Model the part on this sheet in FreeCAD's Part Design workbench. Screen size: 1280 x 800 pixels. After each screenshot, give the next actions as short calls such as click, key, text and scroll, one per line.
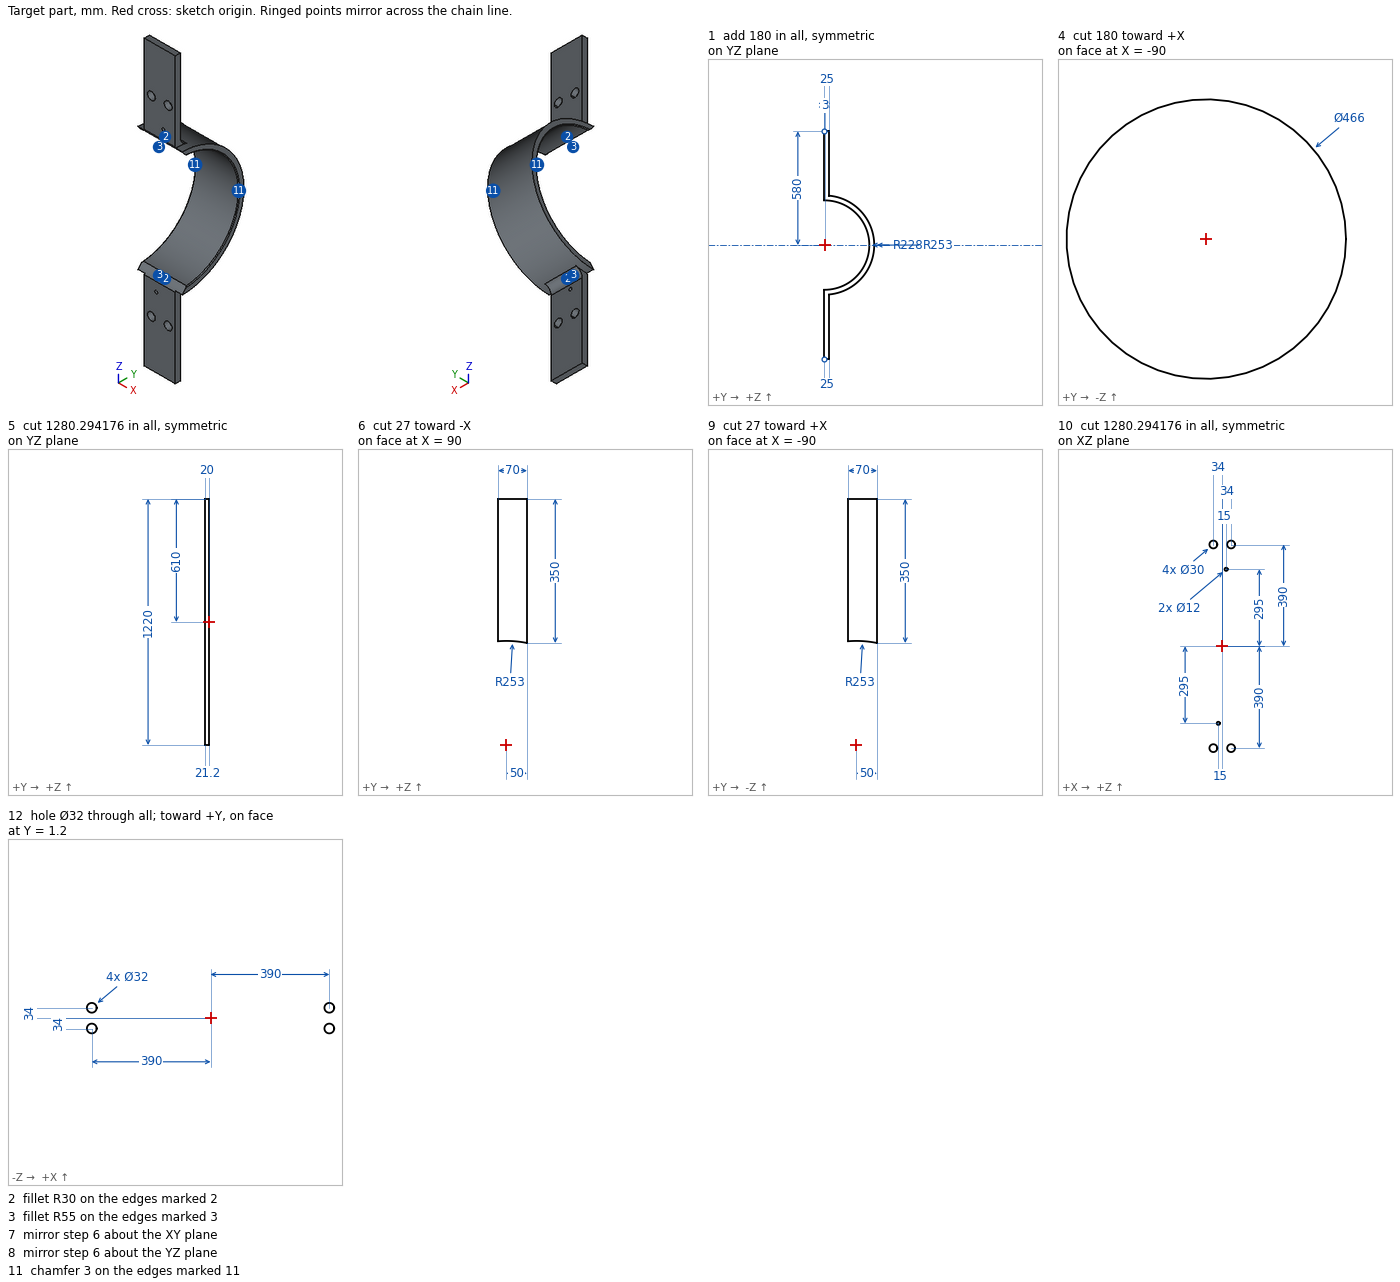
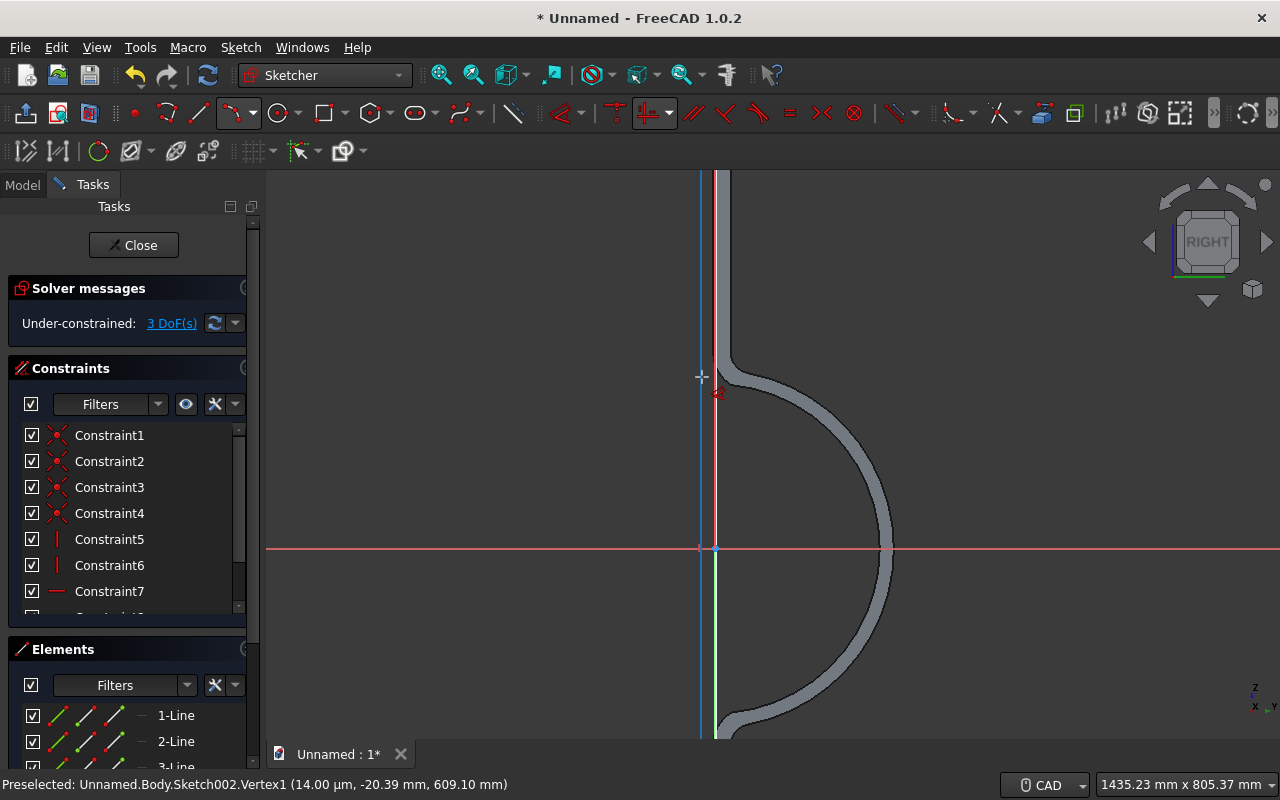
click(701, 377)
click(667, 454)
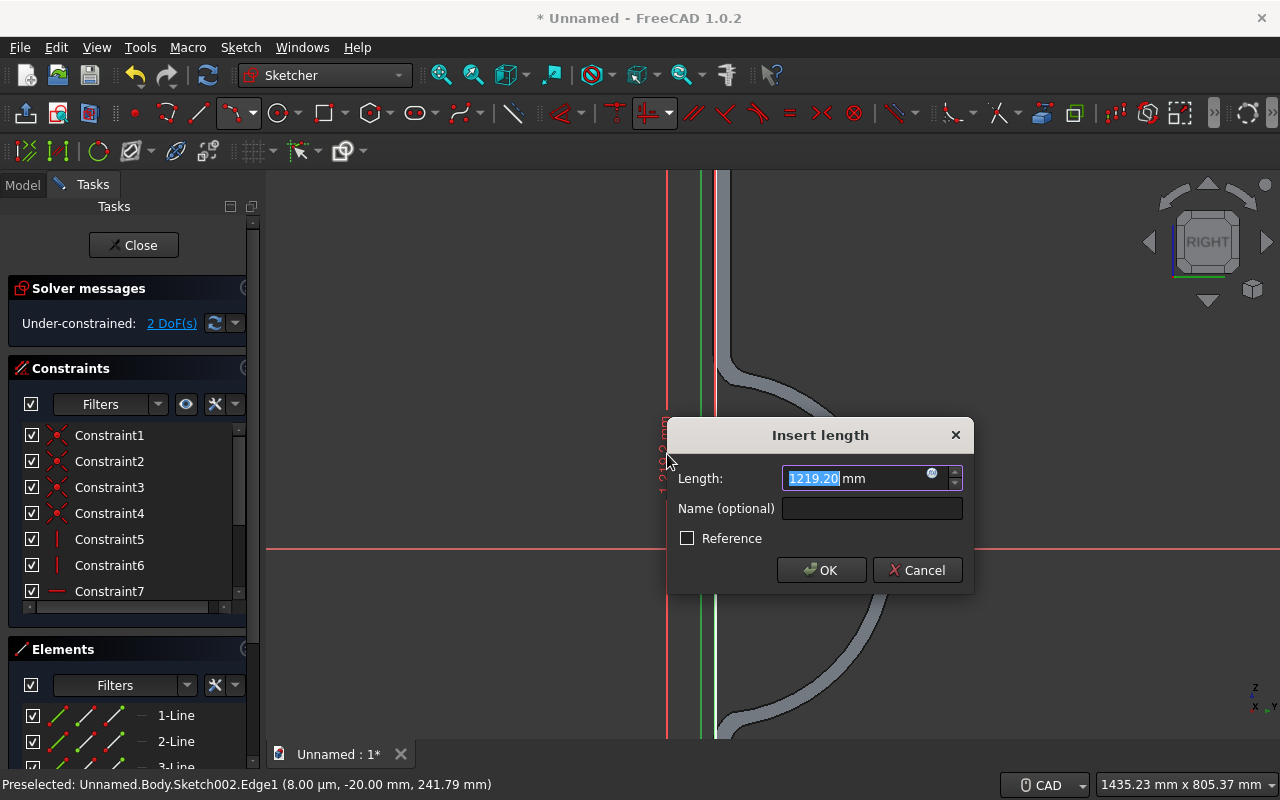
text(1220)
key(Return)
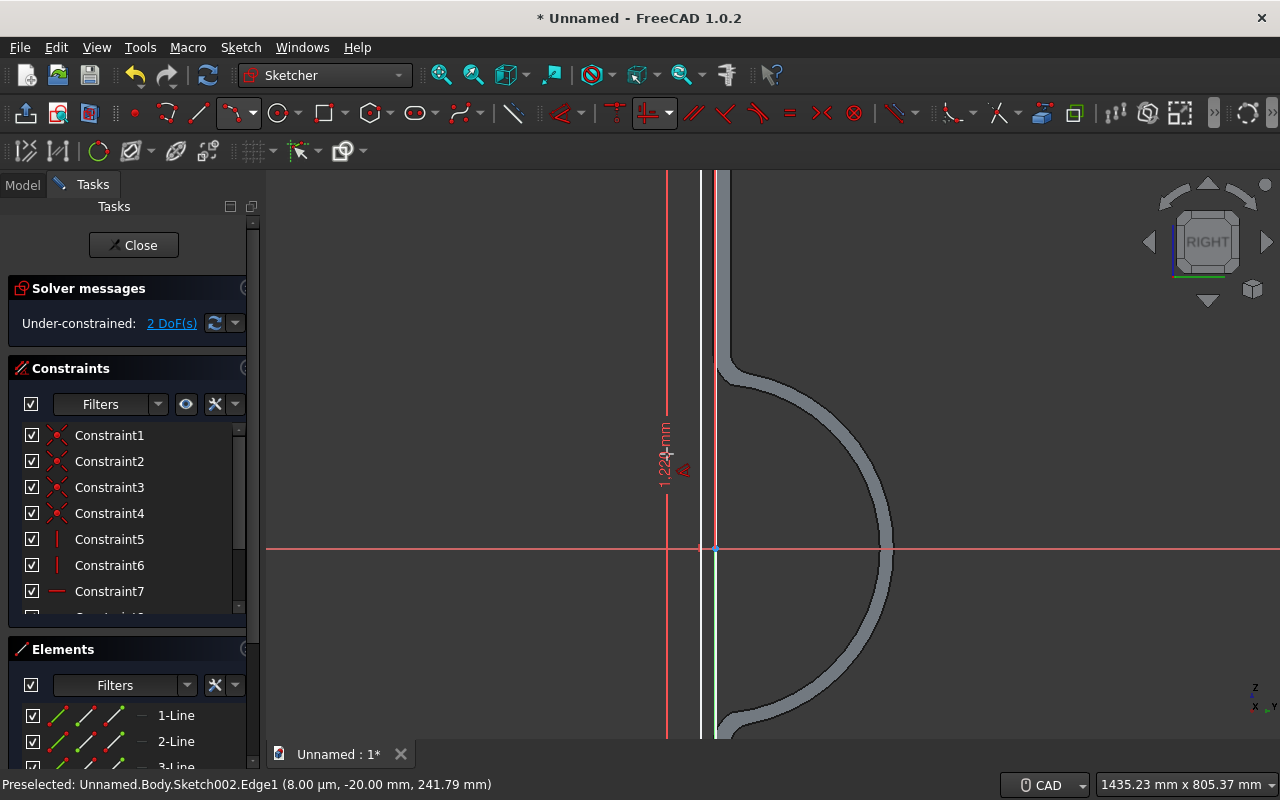
scroll(701, 378, down, 4)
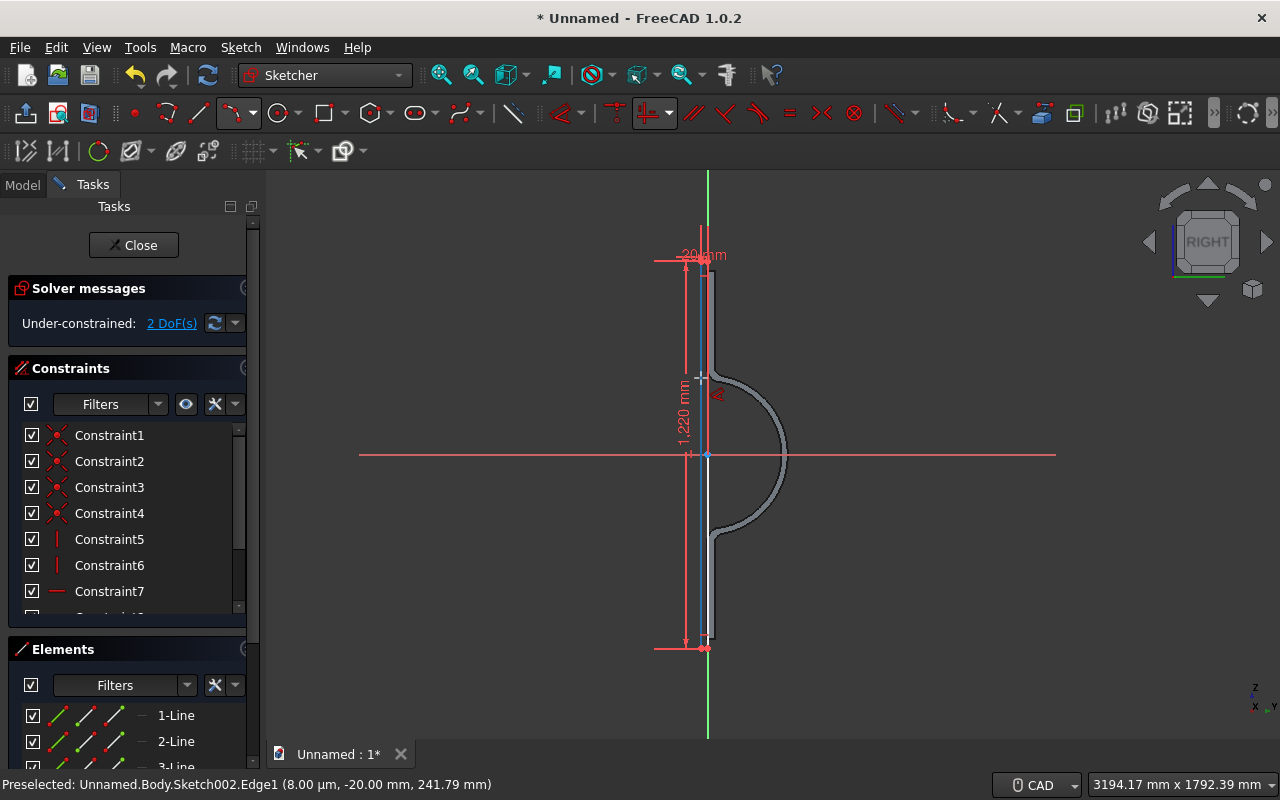
scroll(705, 649, up, 9)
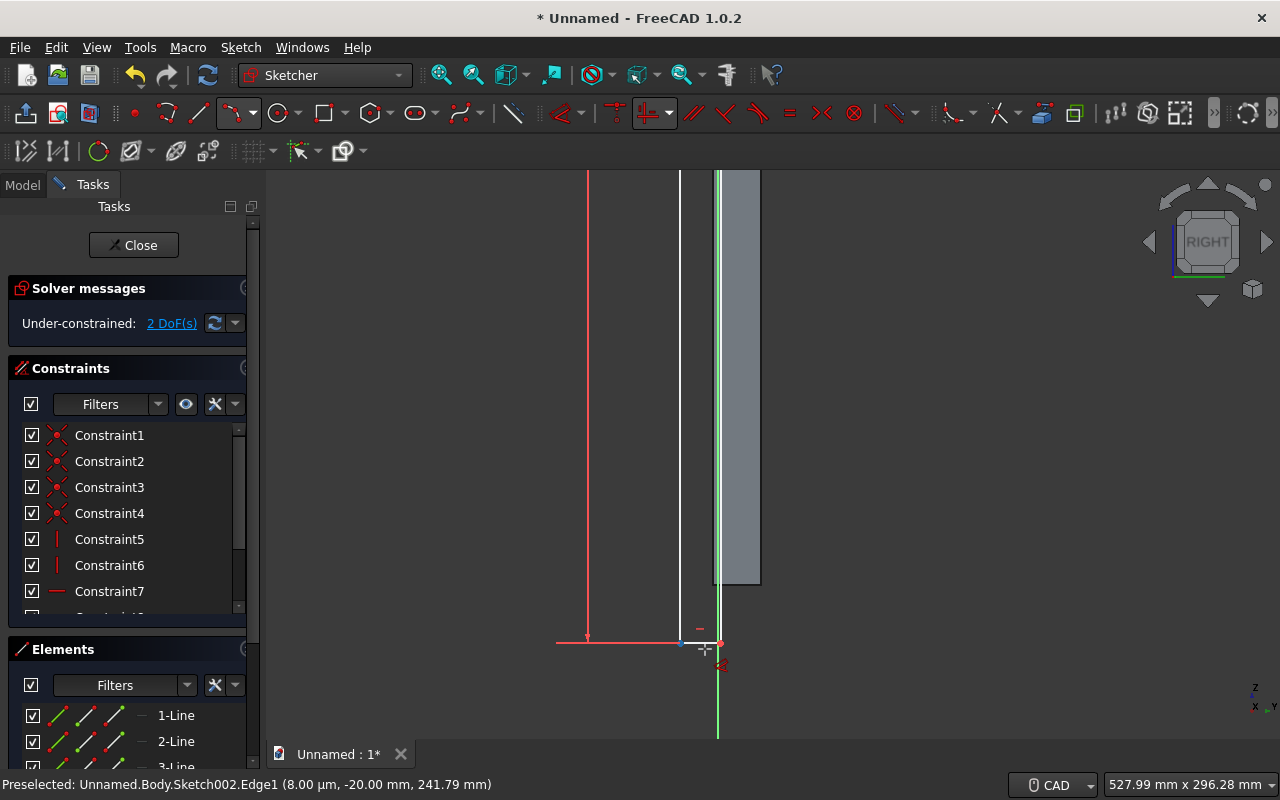
click(700, 643)
click(700, 677)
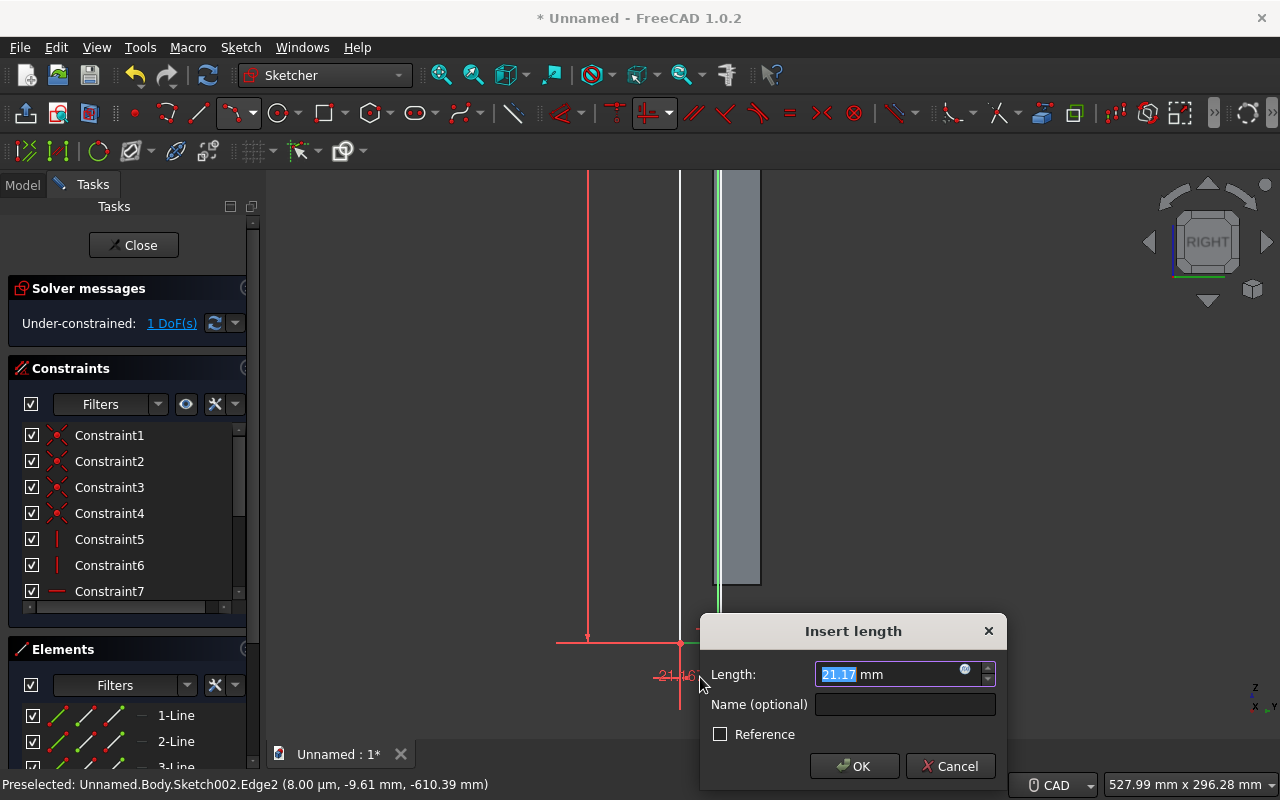
text(21.2)
key(Return)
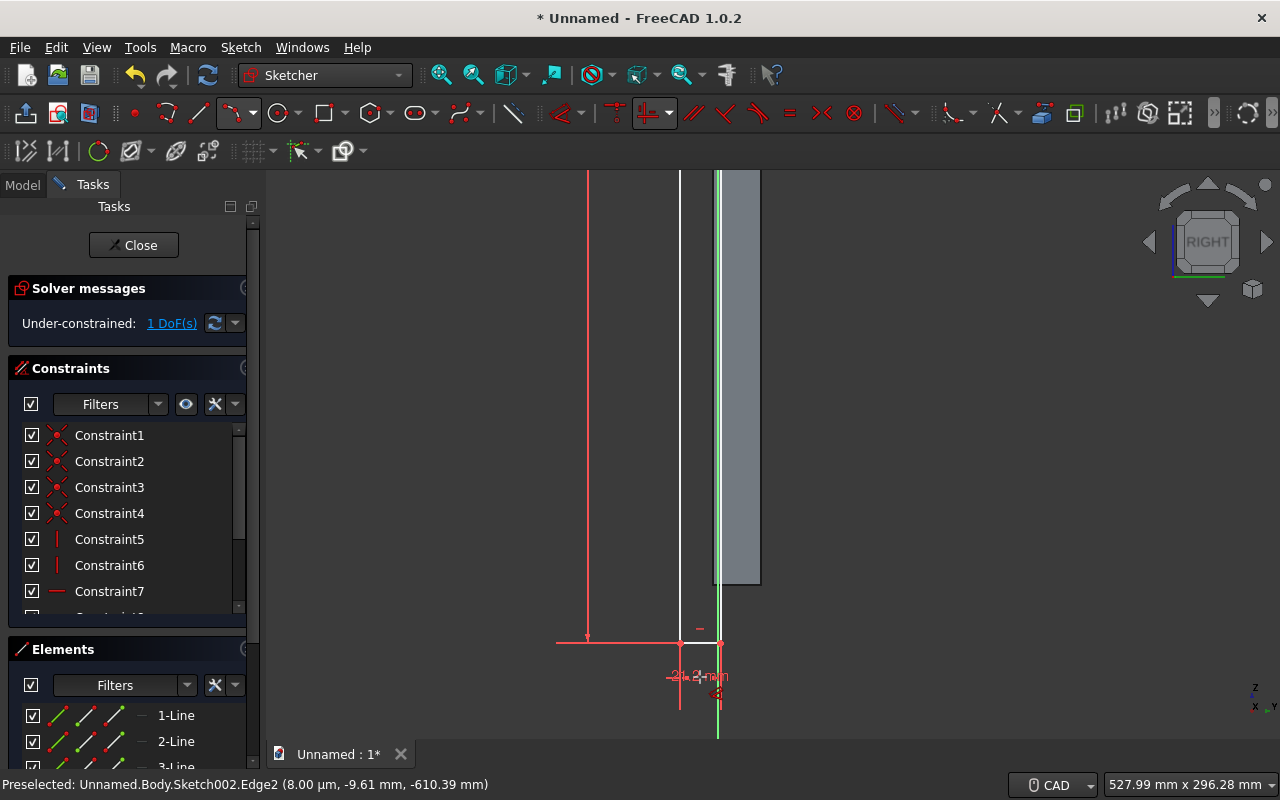
scroll(705, 649, down, 9)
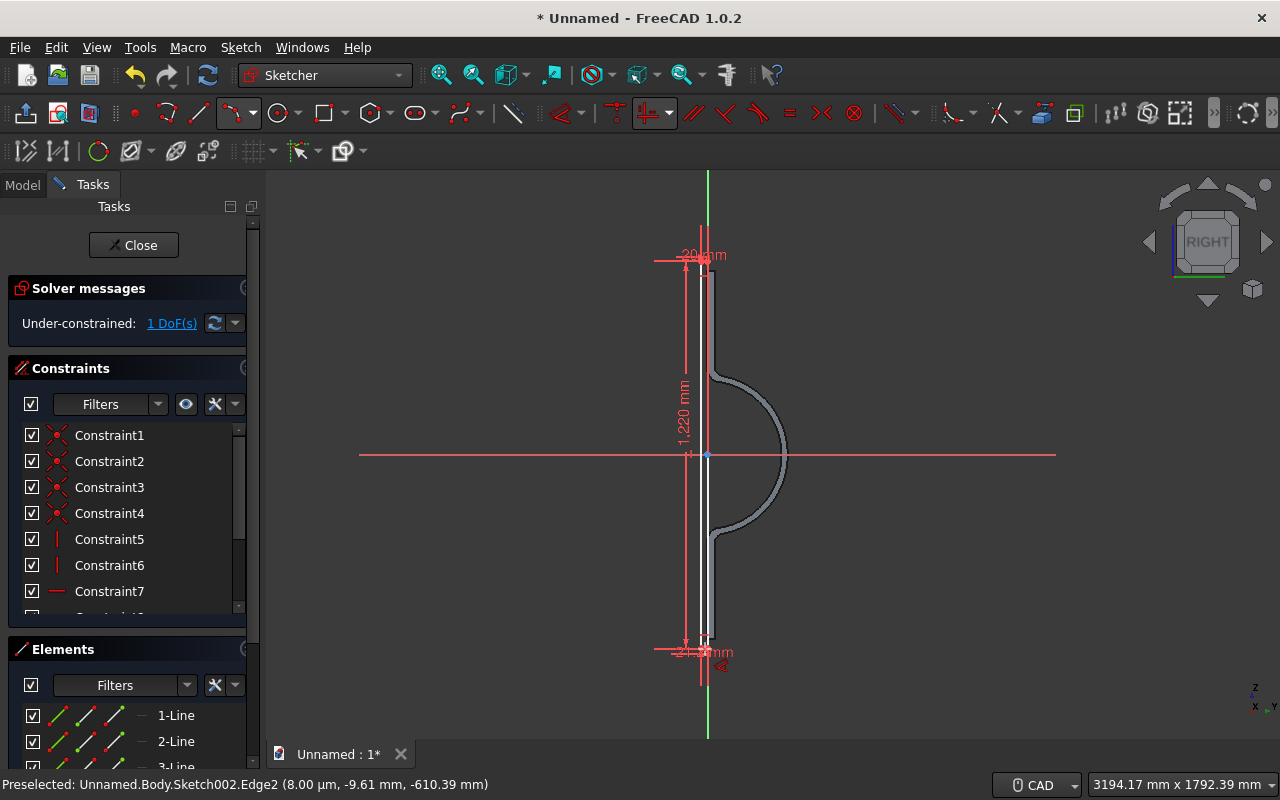
scroll(701, 261, up, 3)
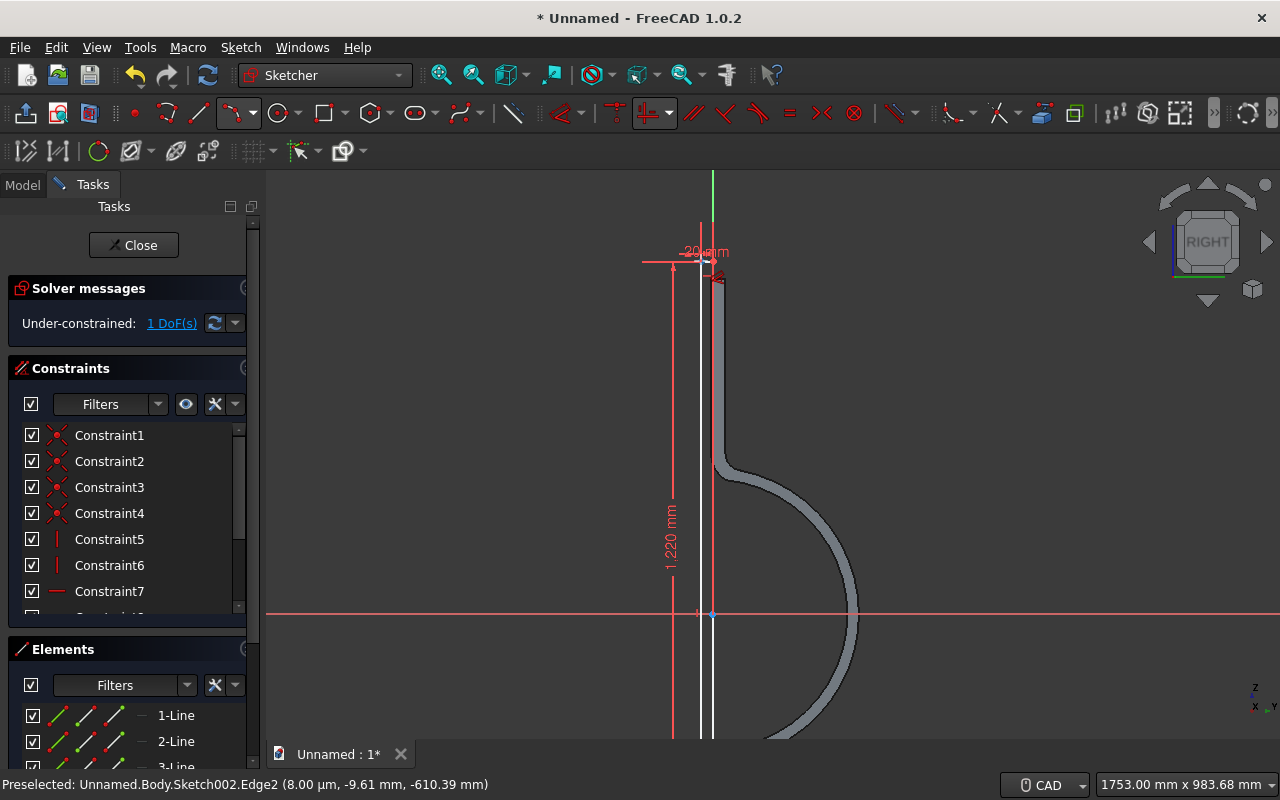
click(701, 262)
click(667, 438)